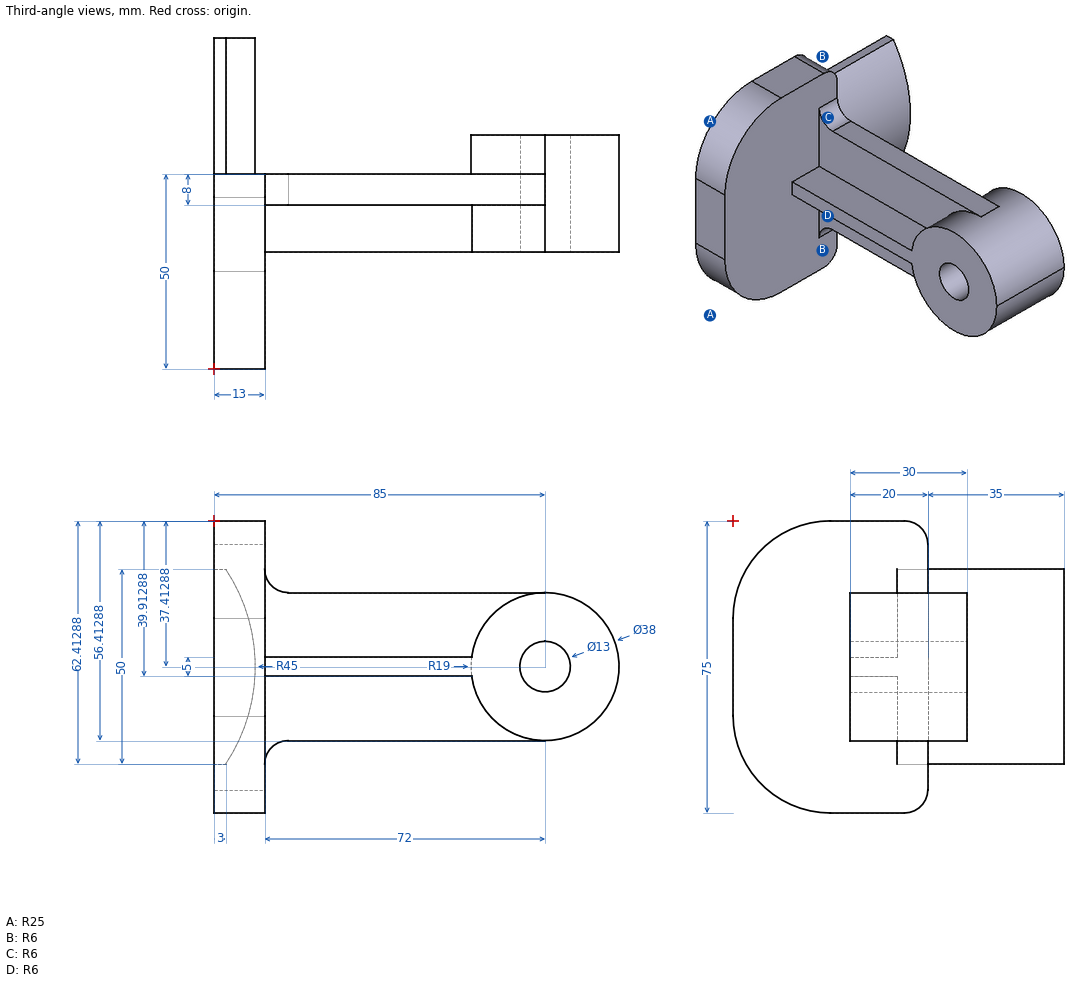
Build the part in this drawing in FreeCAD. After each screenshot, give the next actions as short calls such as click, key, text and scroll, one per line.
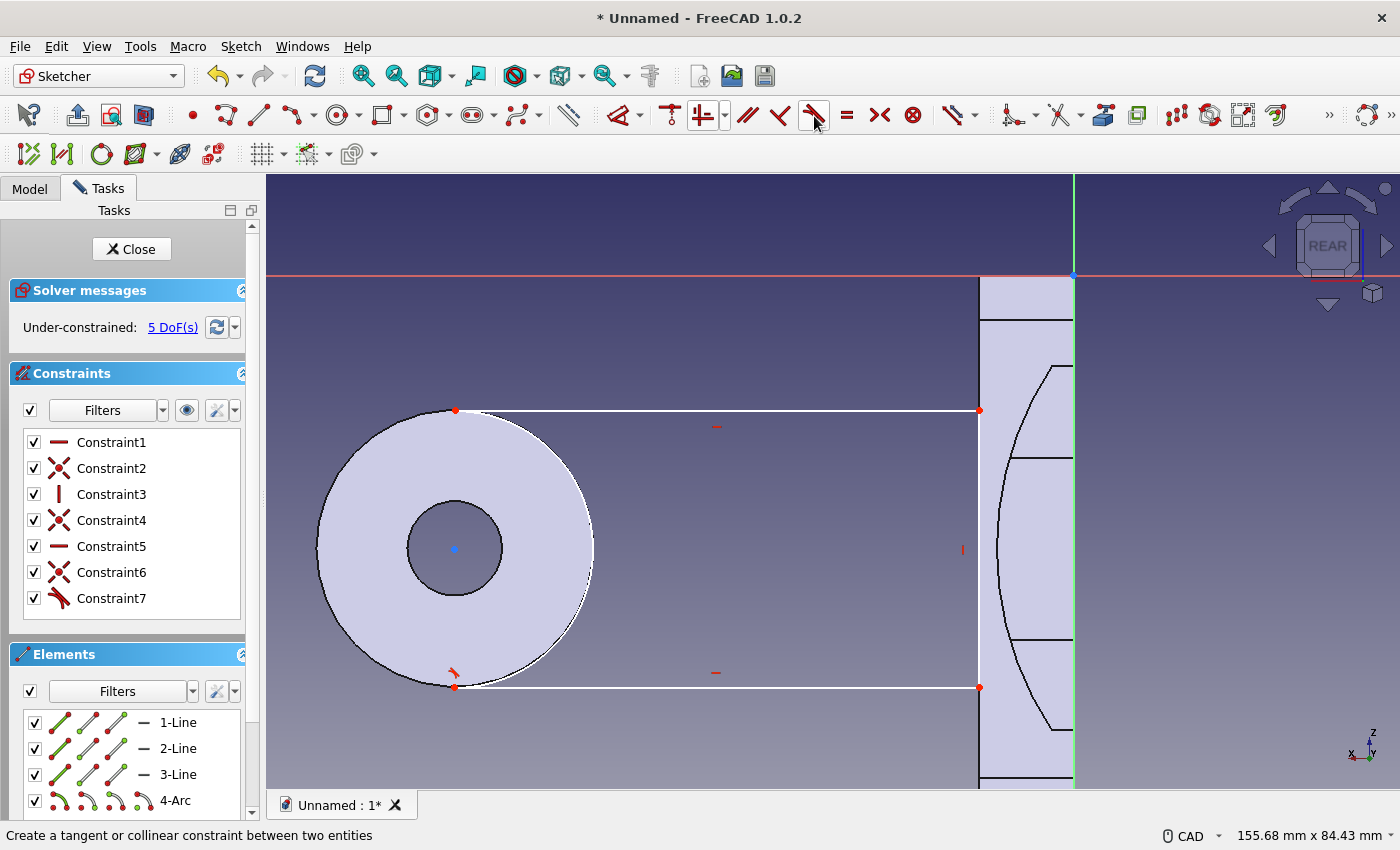
click(822, 411)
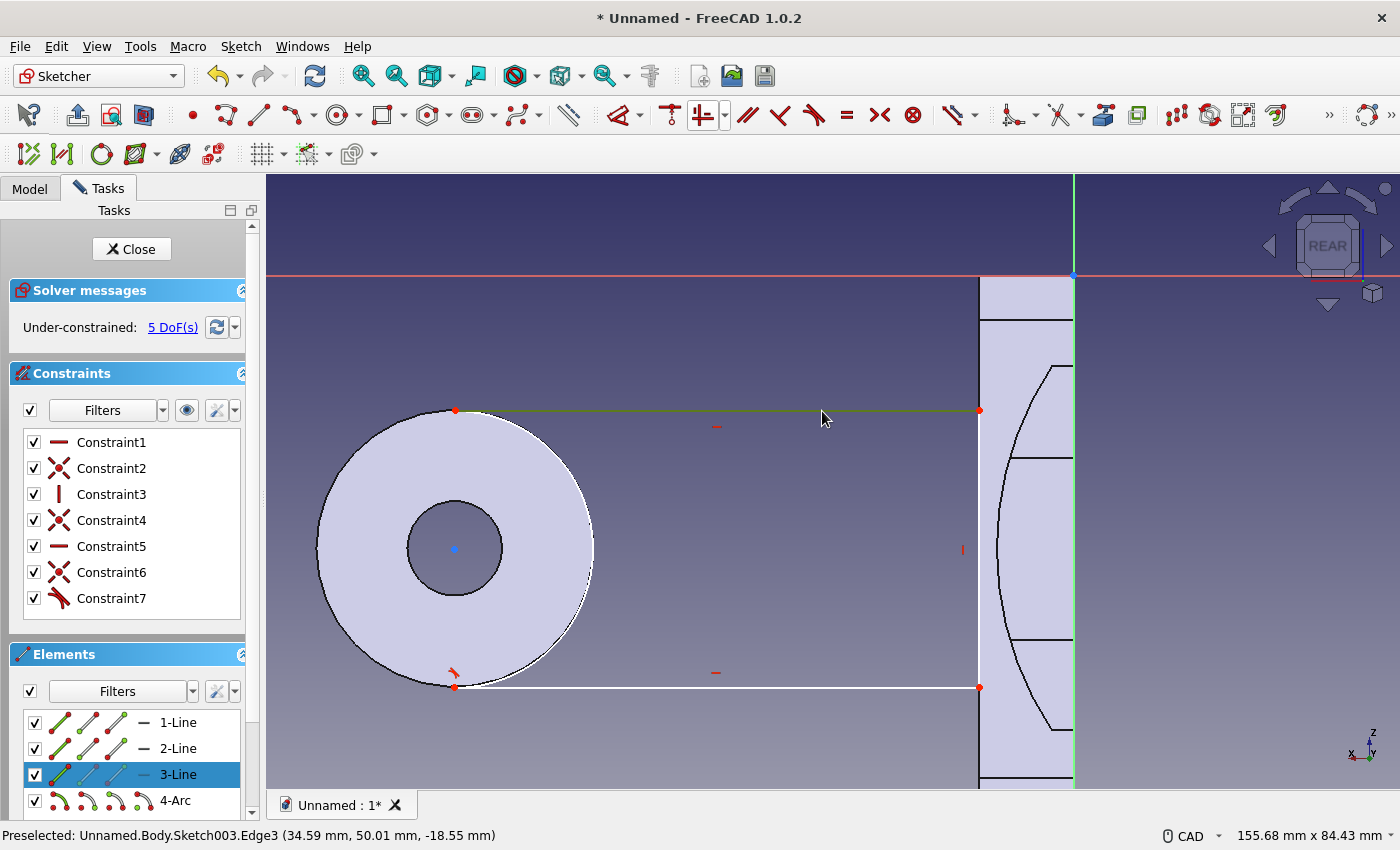
click(566, 631)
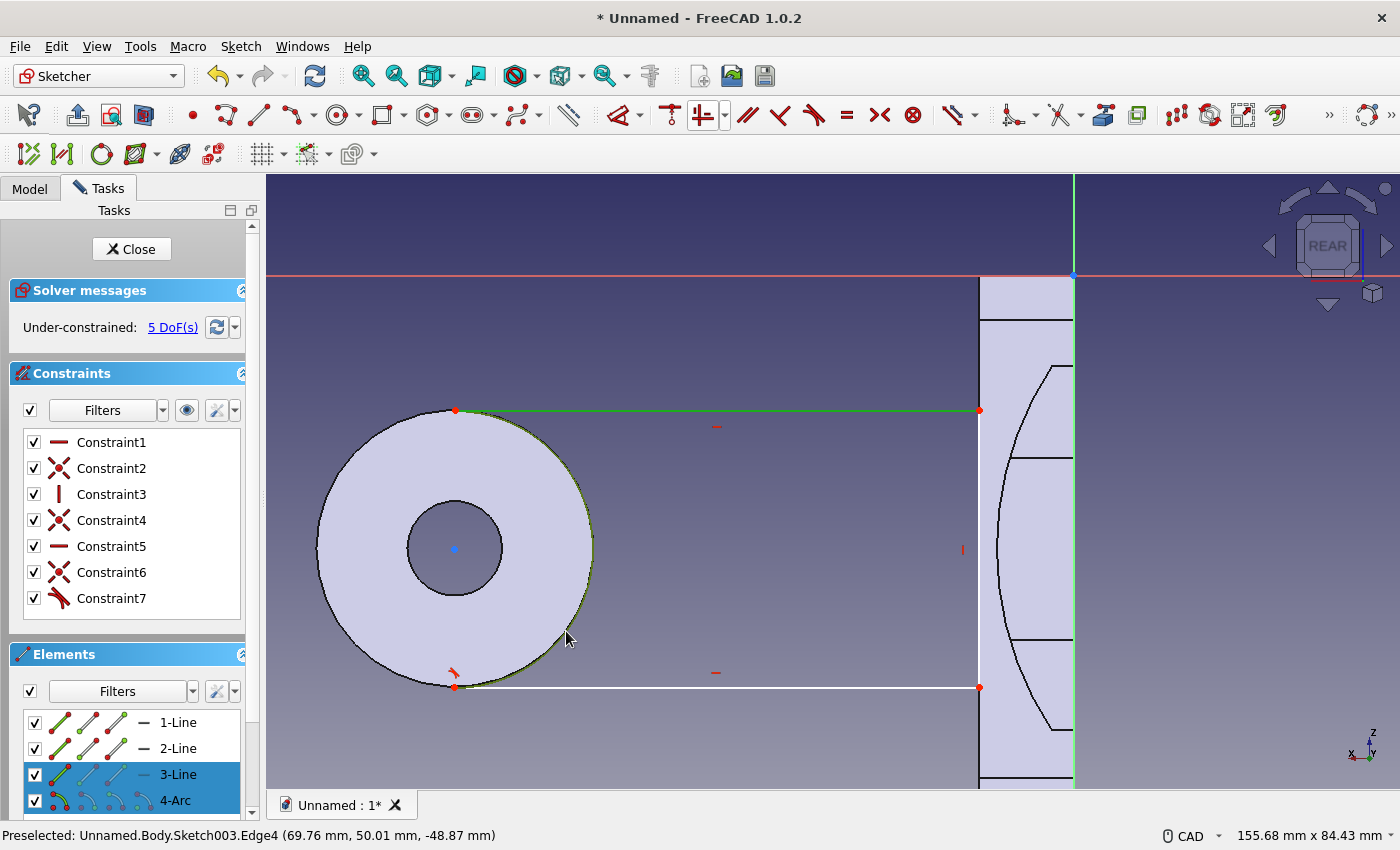
click(814, 116)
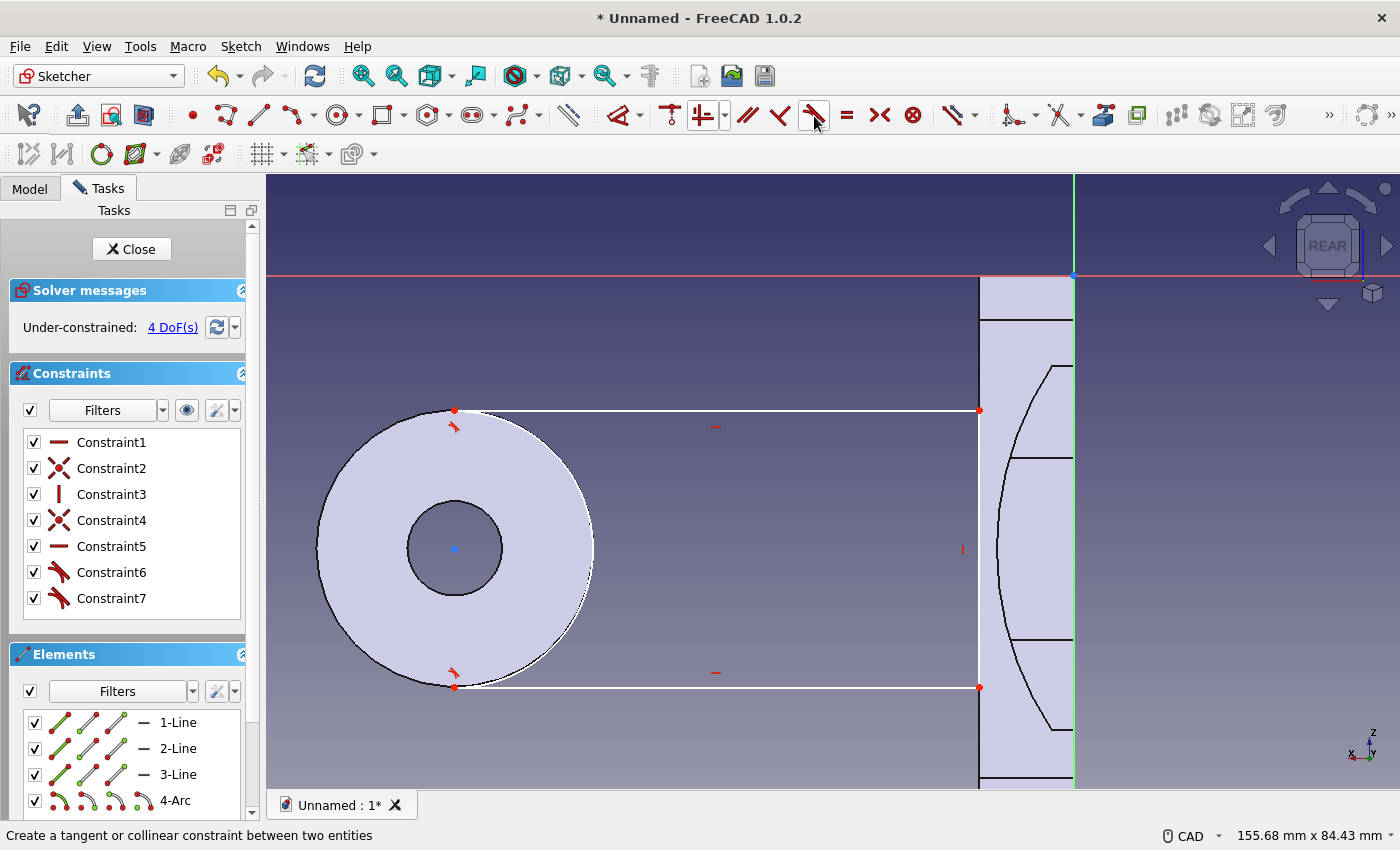
click(618, 116)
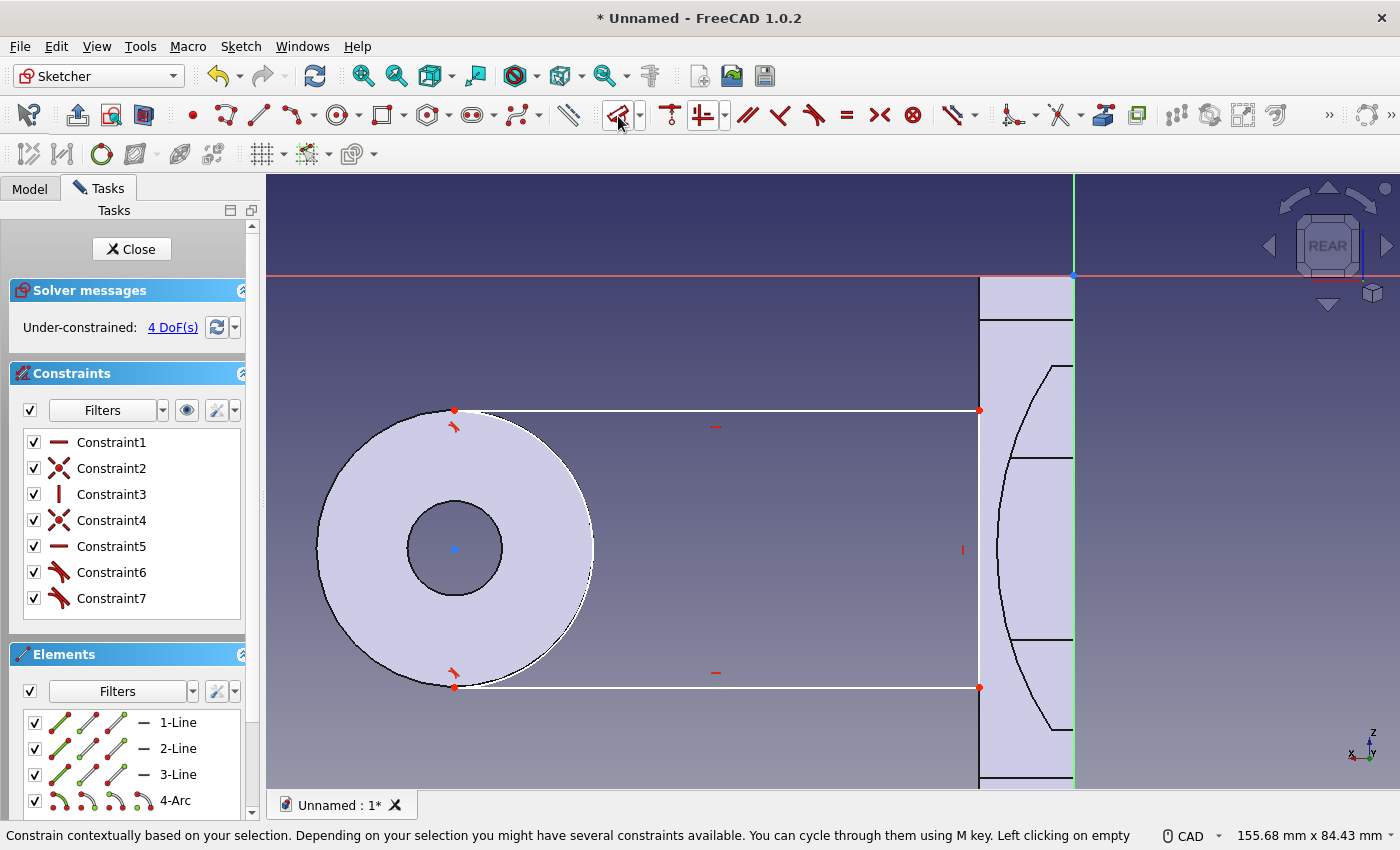
click(567, 631)
click(593, 650)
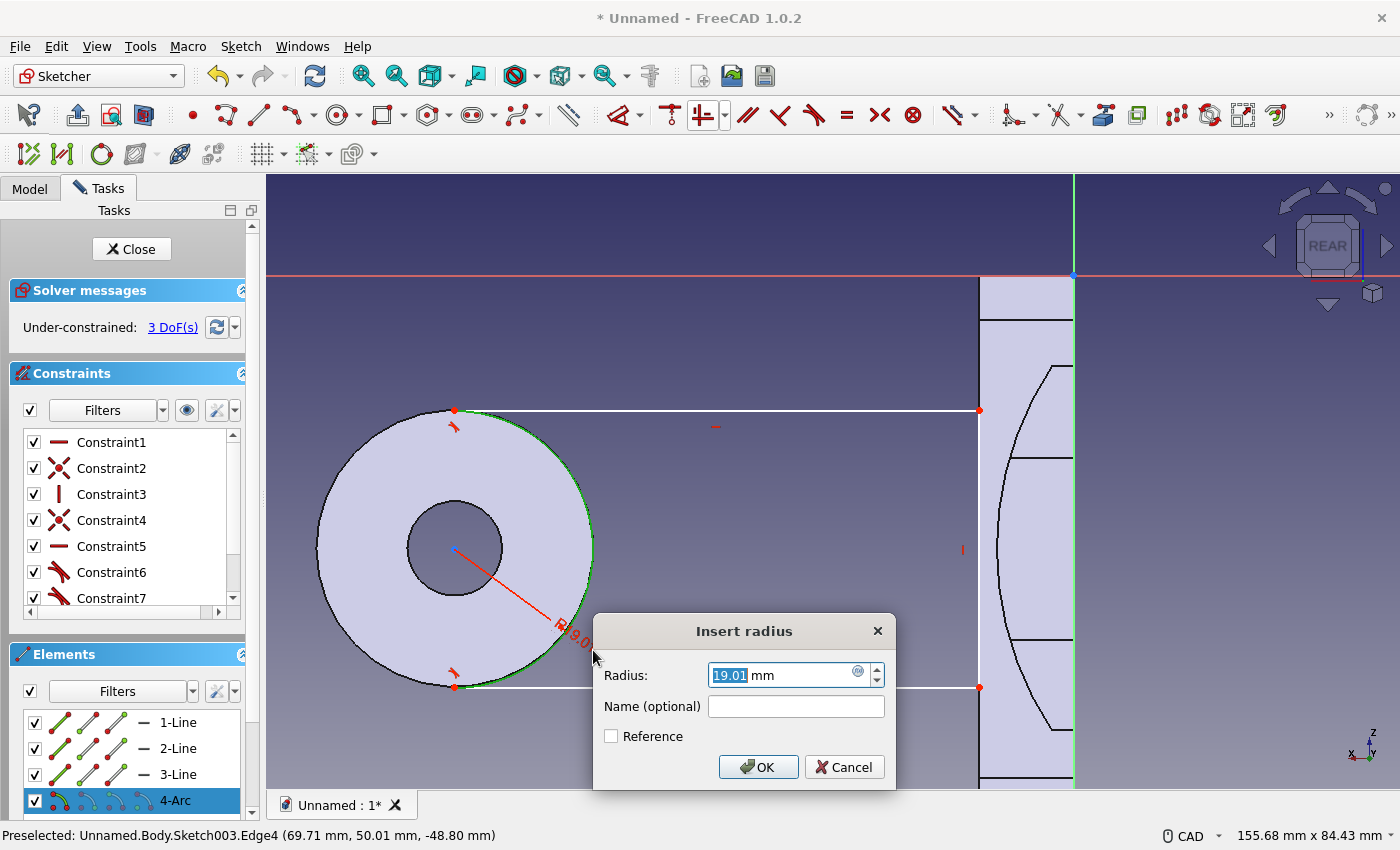
text(19)
key(Return)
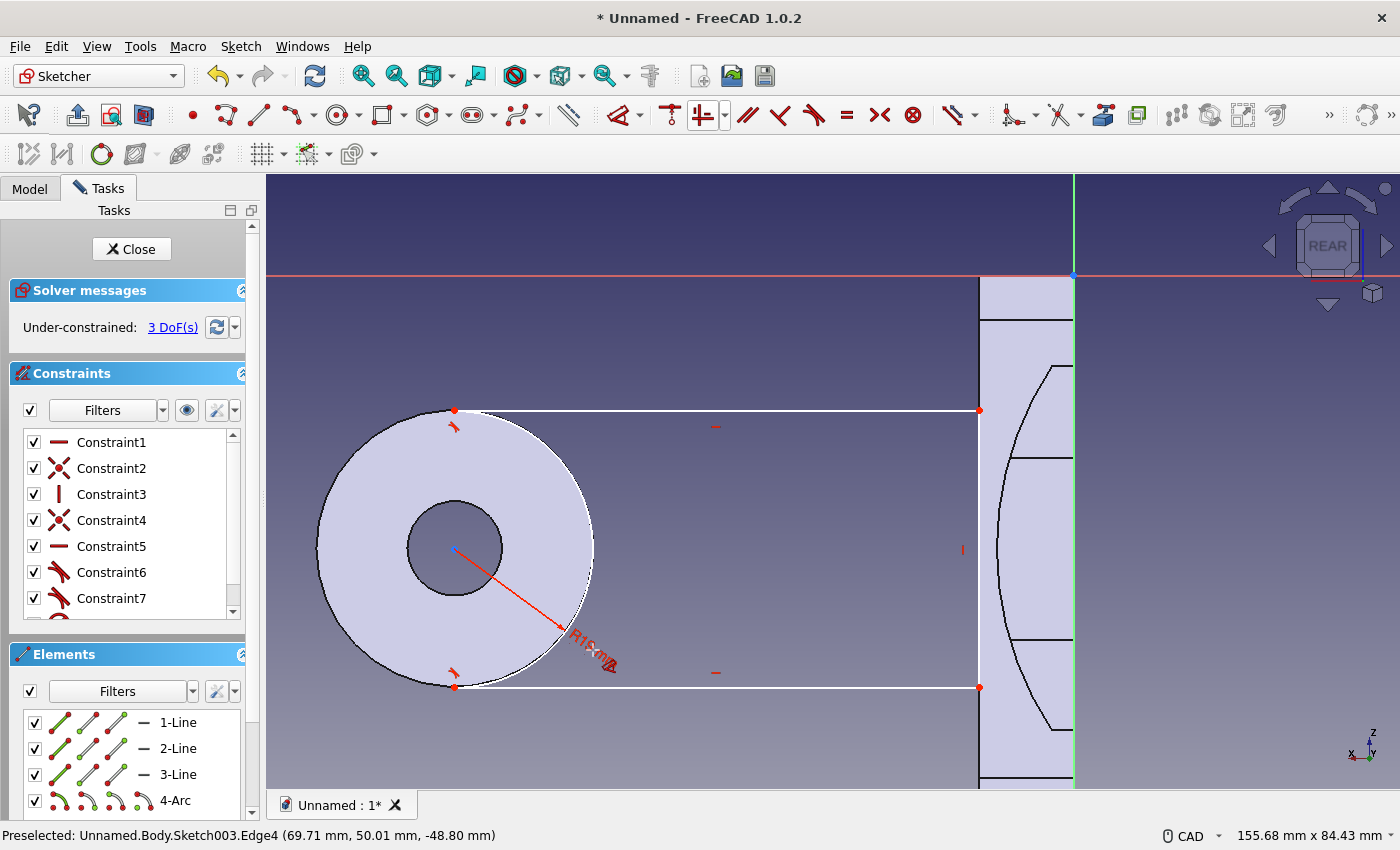
click(612, 688)
click(717, 722)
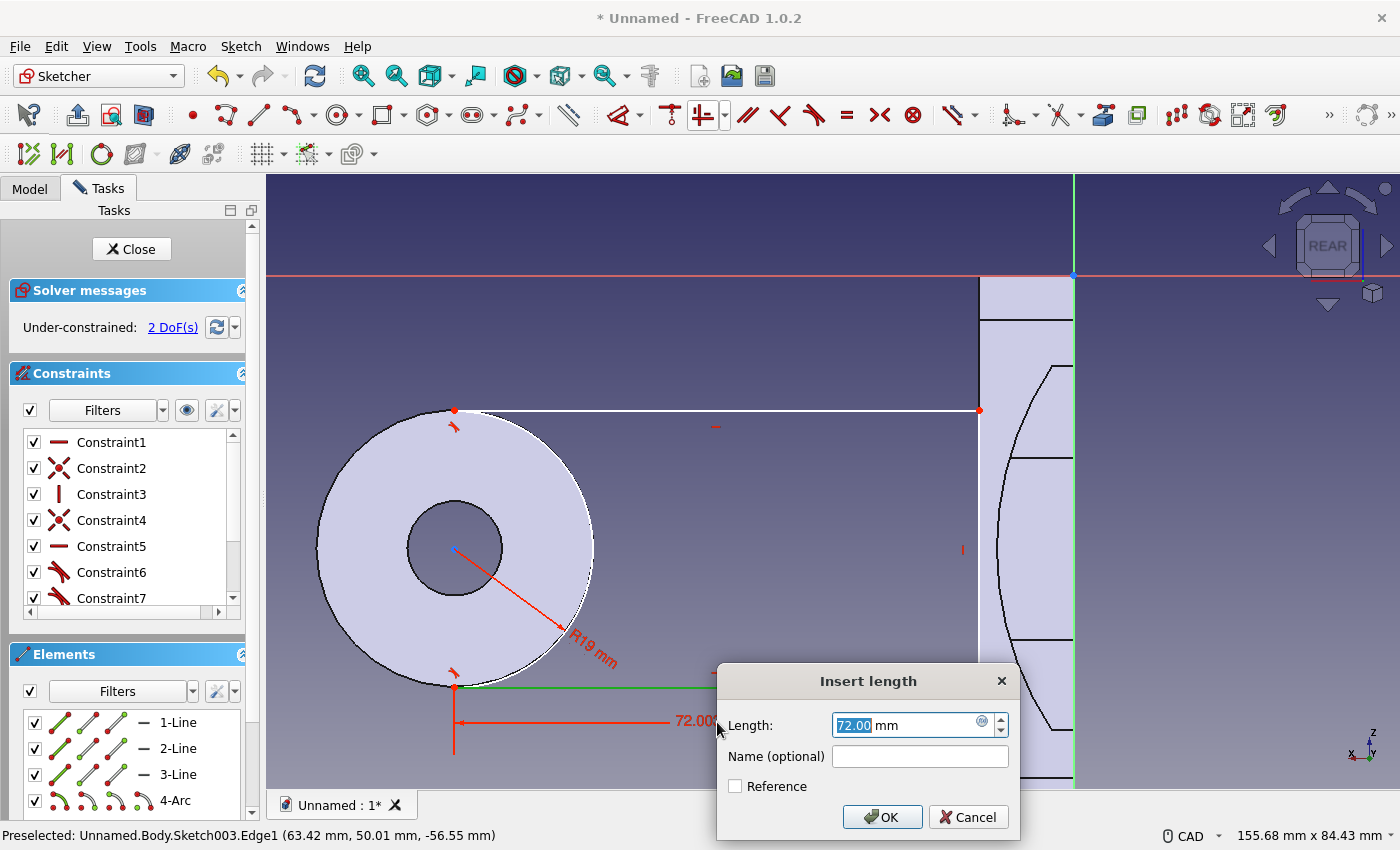
text(72)
key(Return)